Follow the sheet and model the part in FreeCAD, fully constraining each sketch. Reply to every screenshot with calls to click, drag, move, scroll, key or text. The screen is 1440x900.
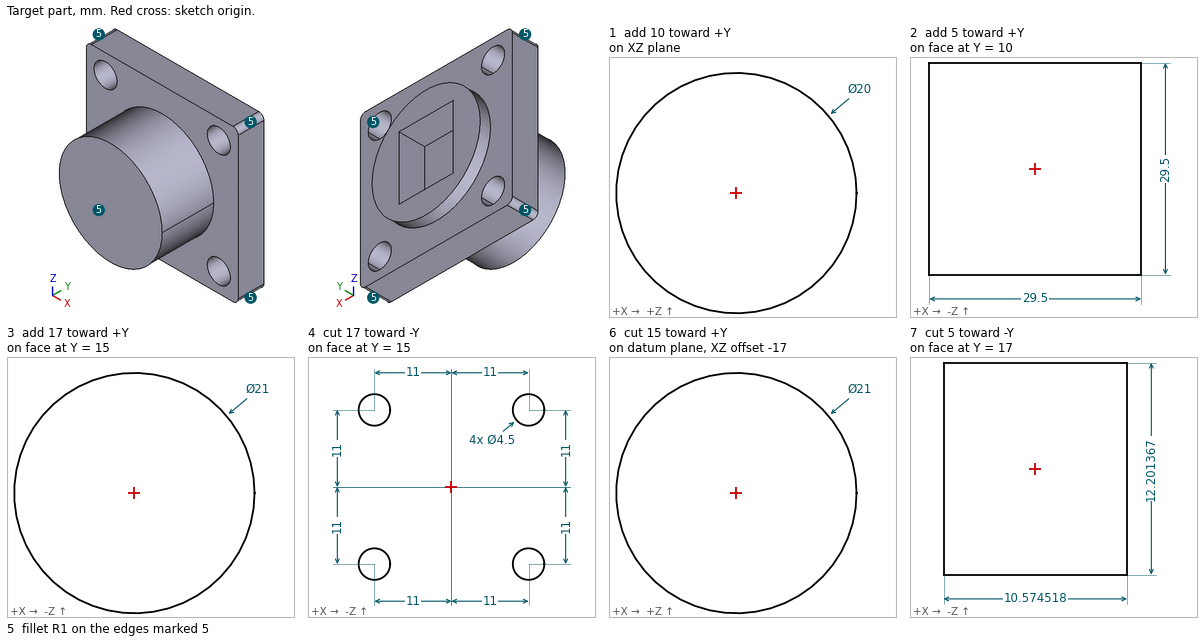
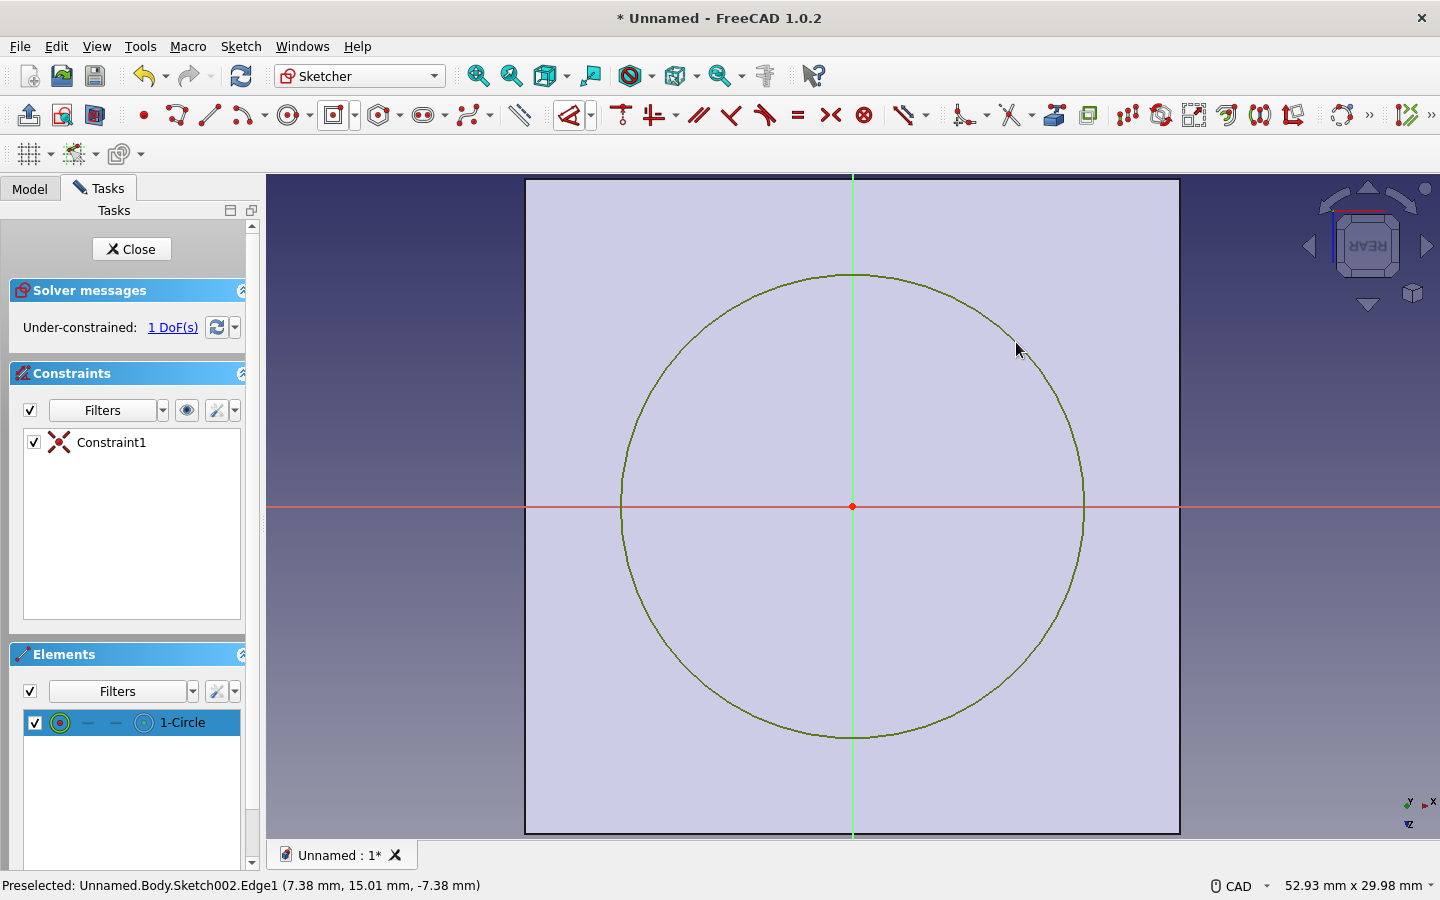
key(k)
key(o)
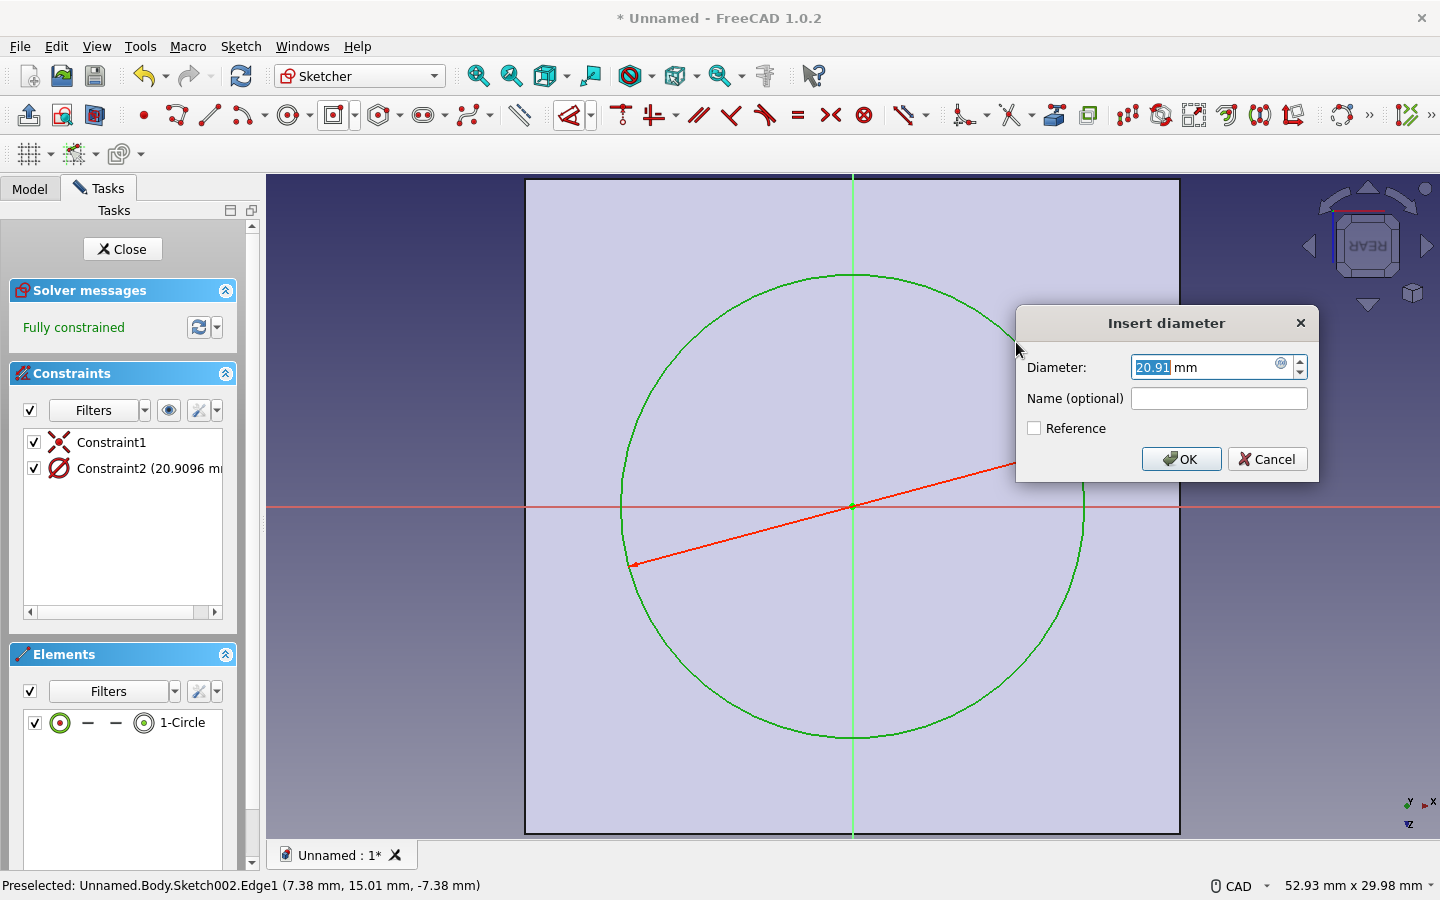
text(21)
key(Return)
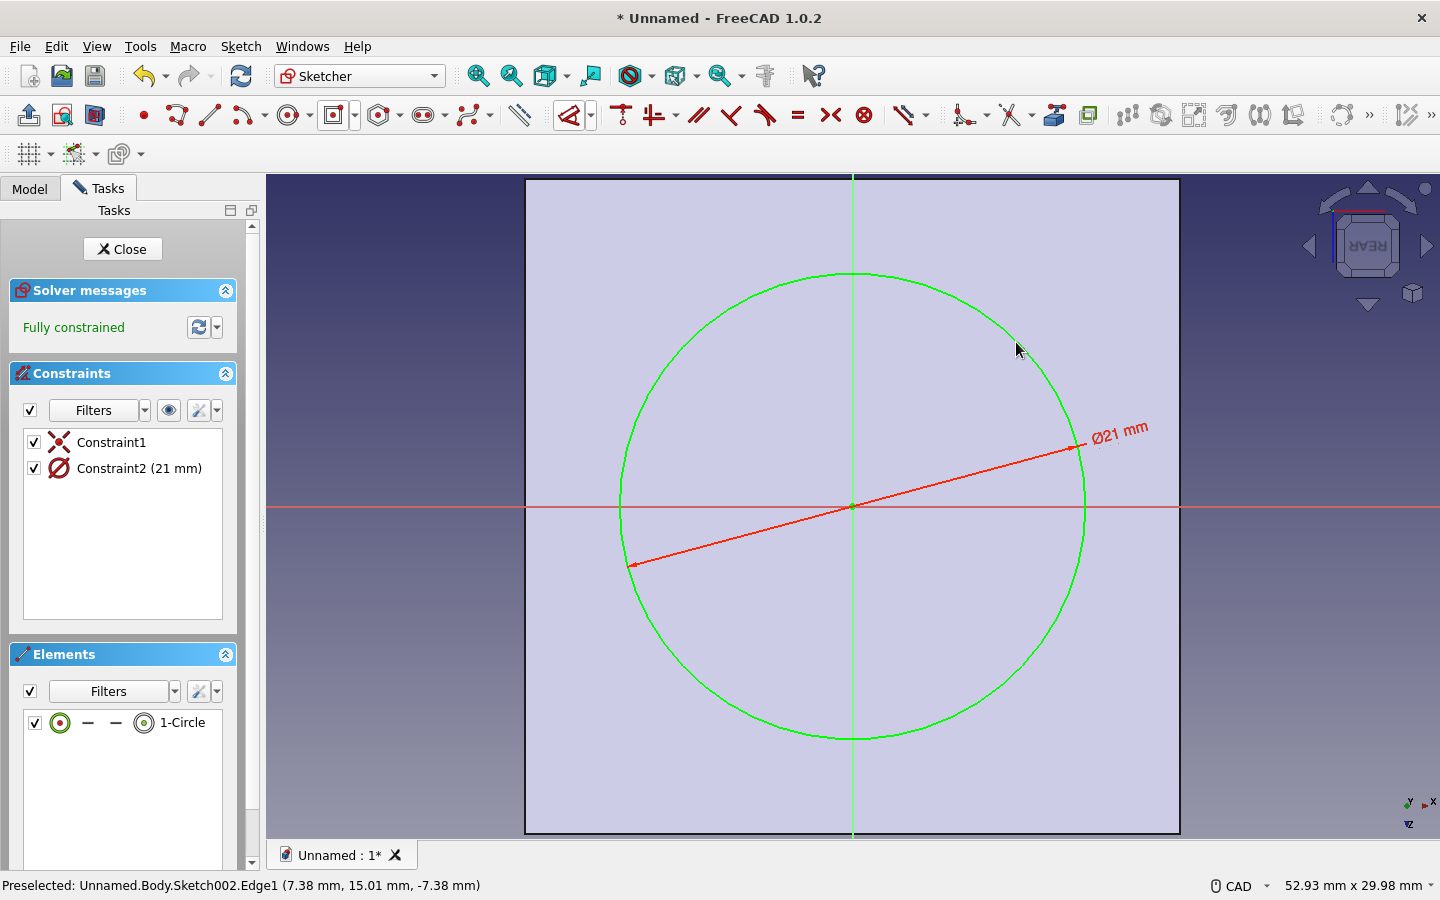
click(123, 249)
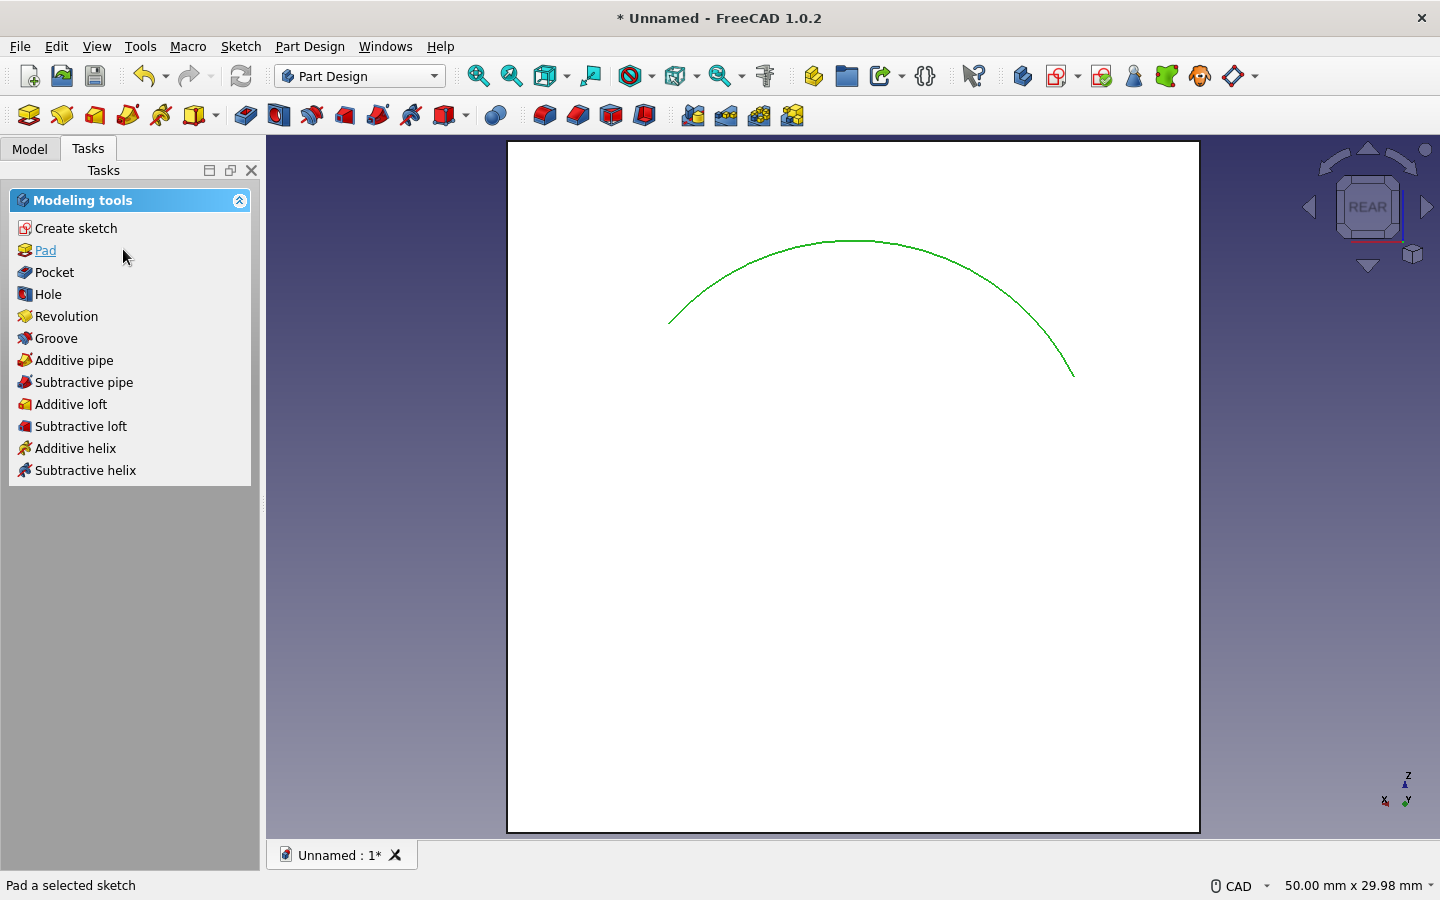
click(29, 116)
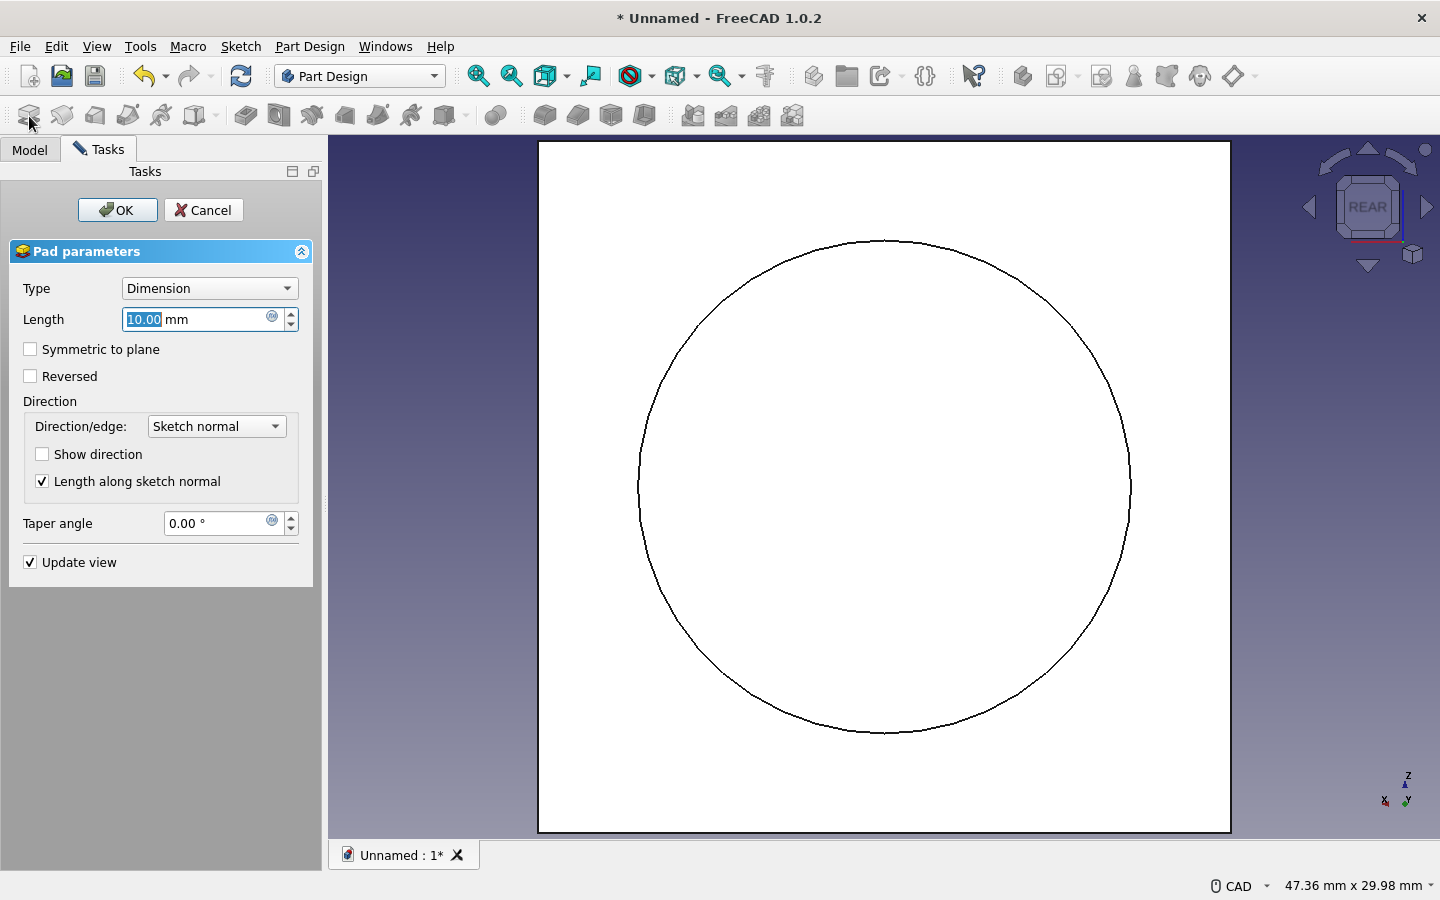
text(17)
key(Tab)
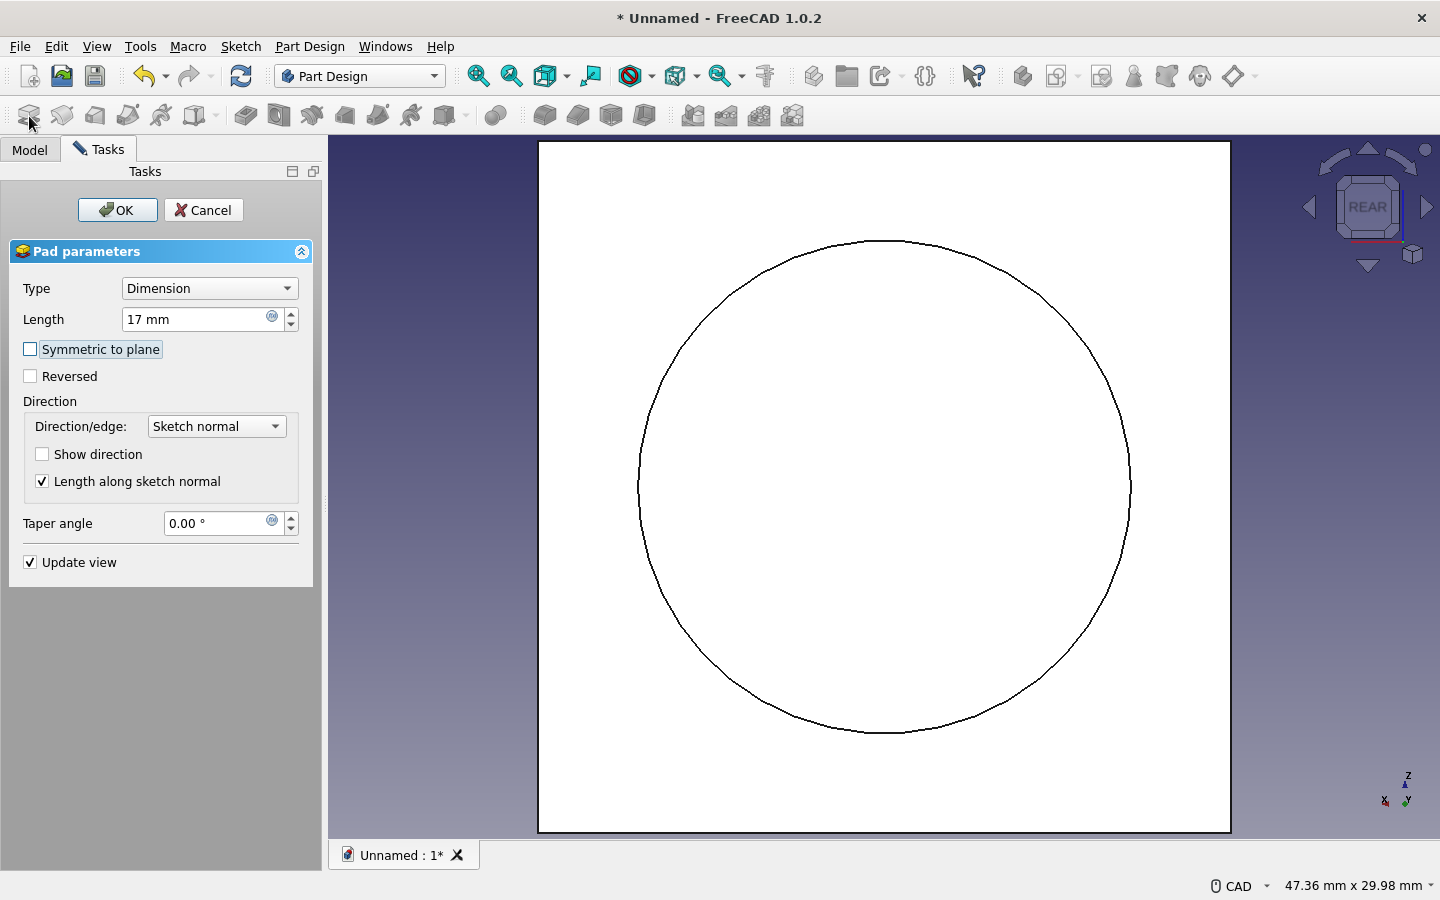
click(118, 210)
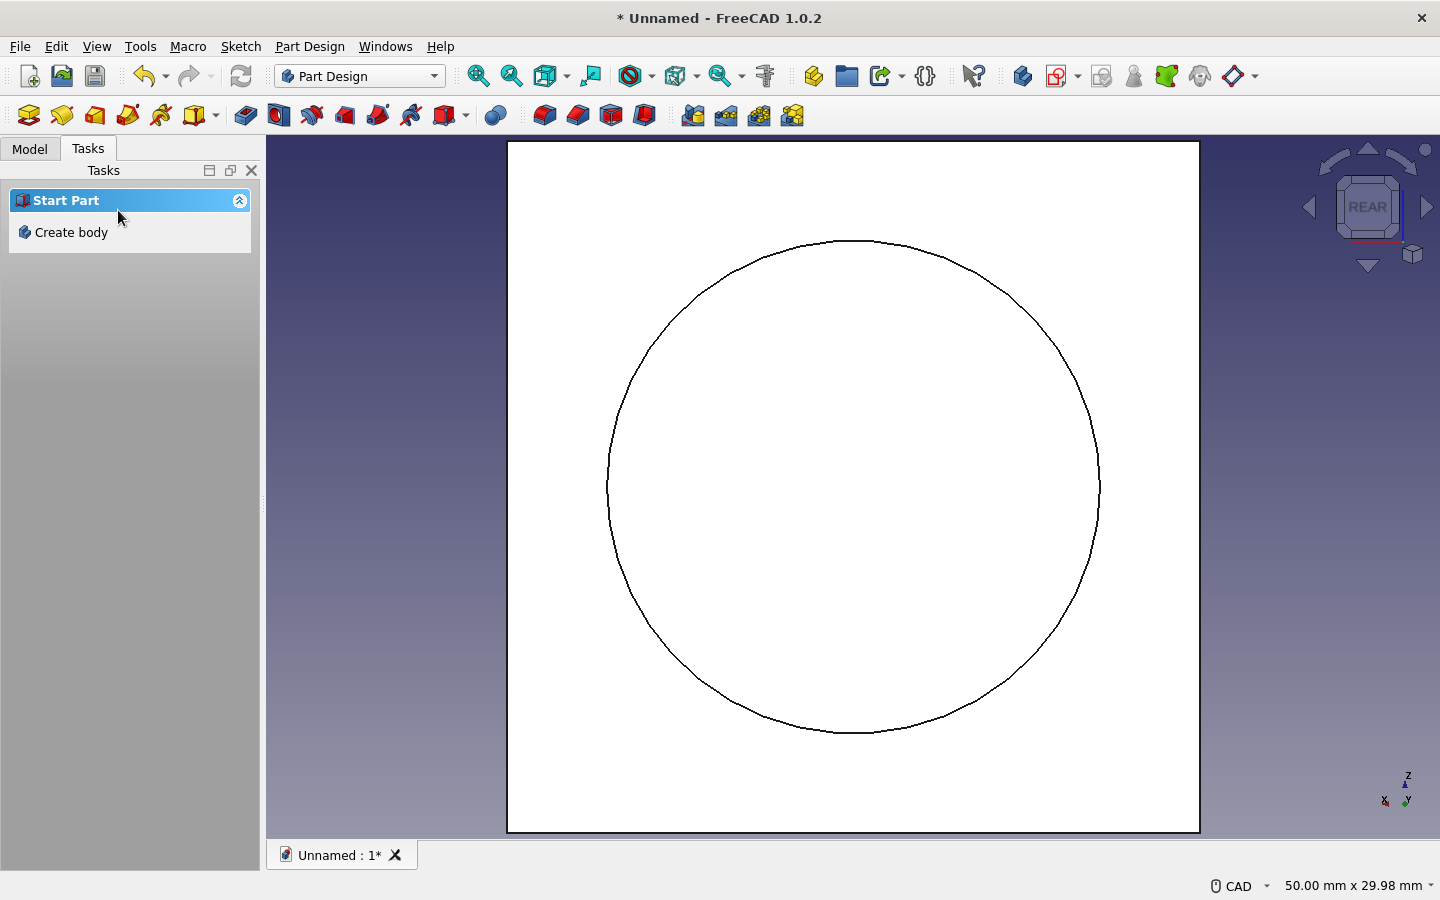
click(557, 783)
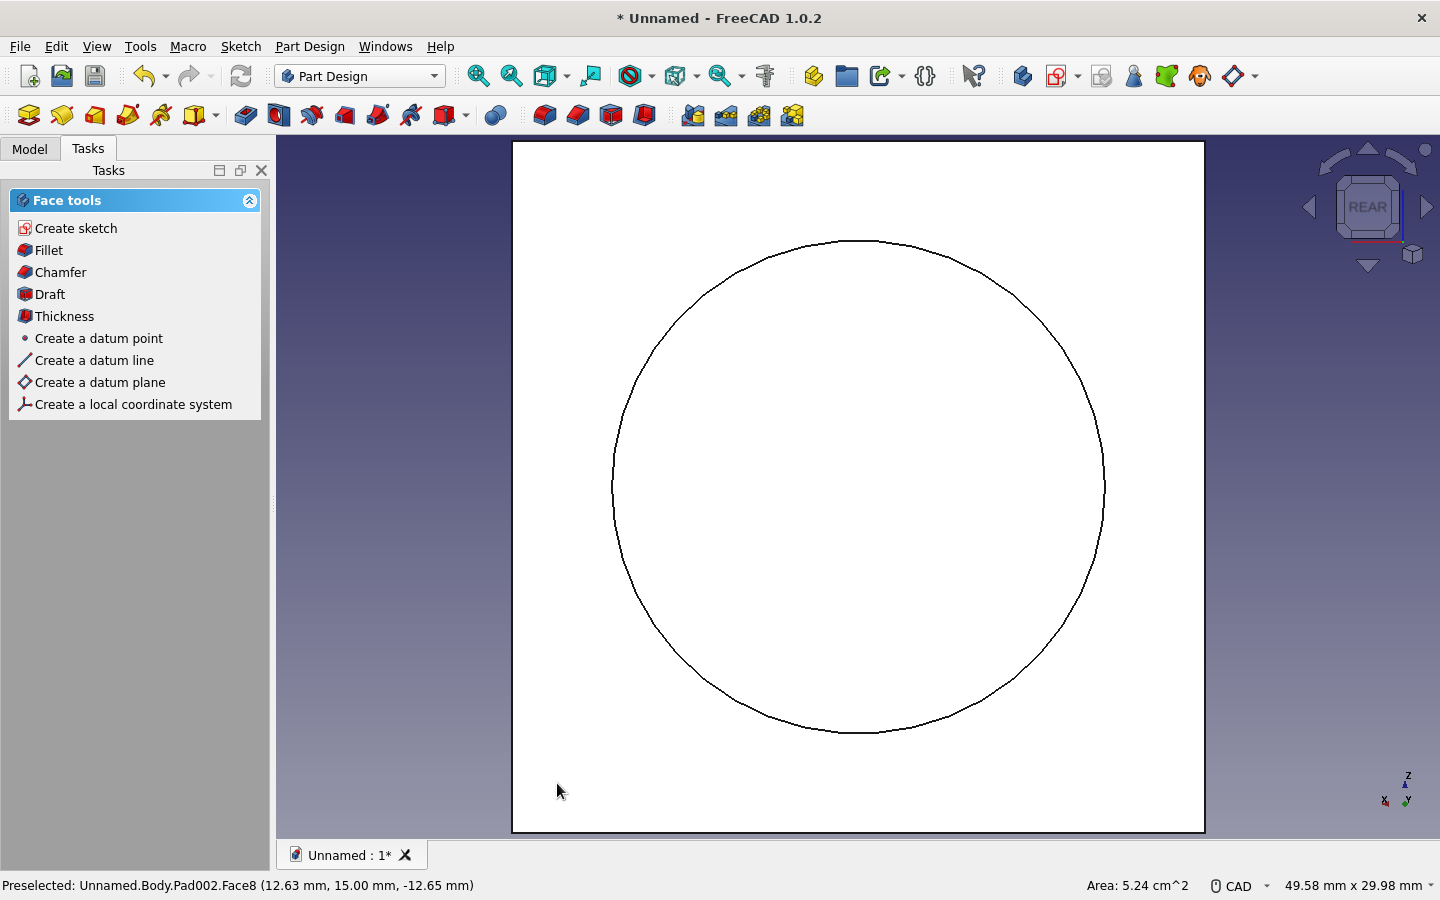
click(1056, 76)